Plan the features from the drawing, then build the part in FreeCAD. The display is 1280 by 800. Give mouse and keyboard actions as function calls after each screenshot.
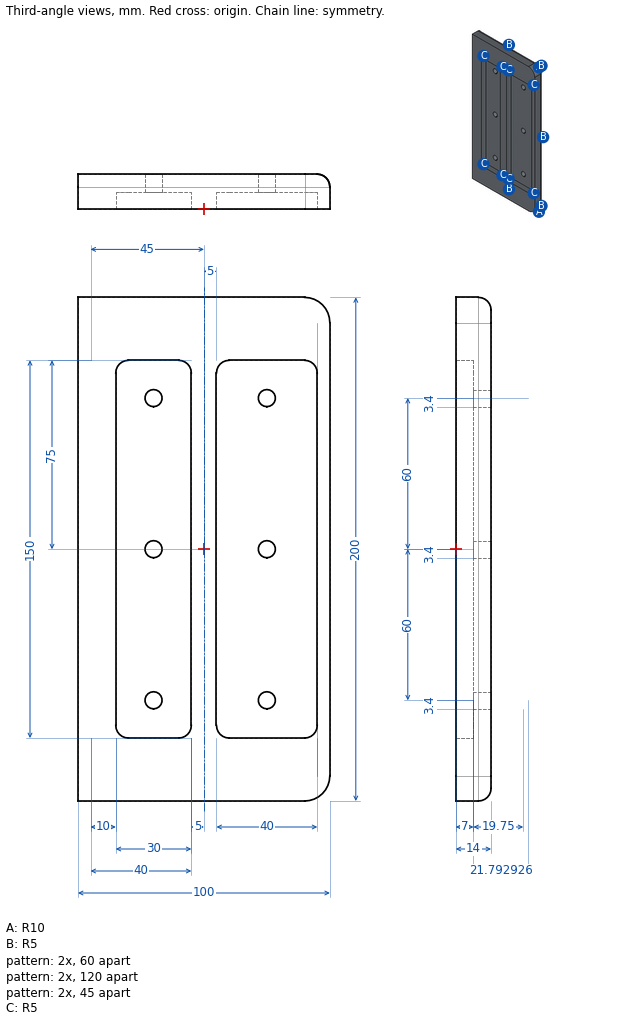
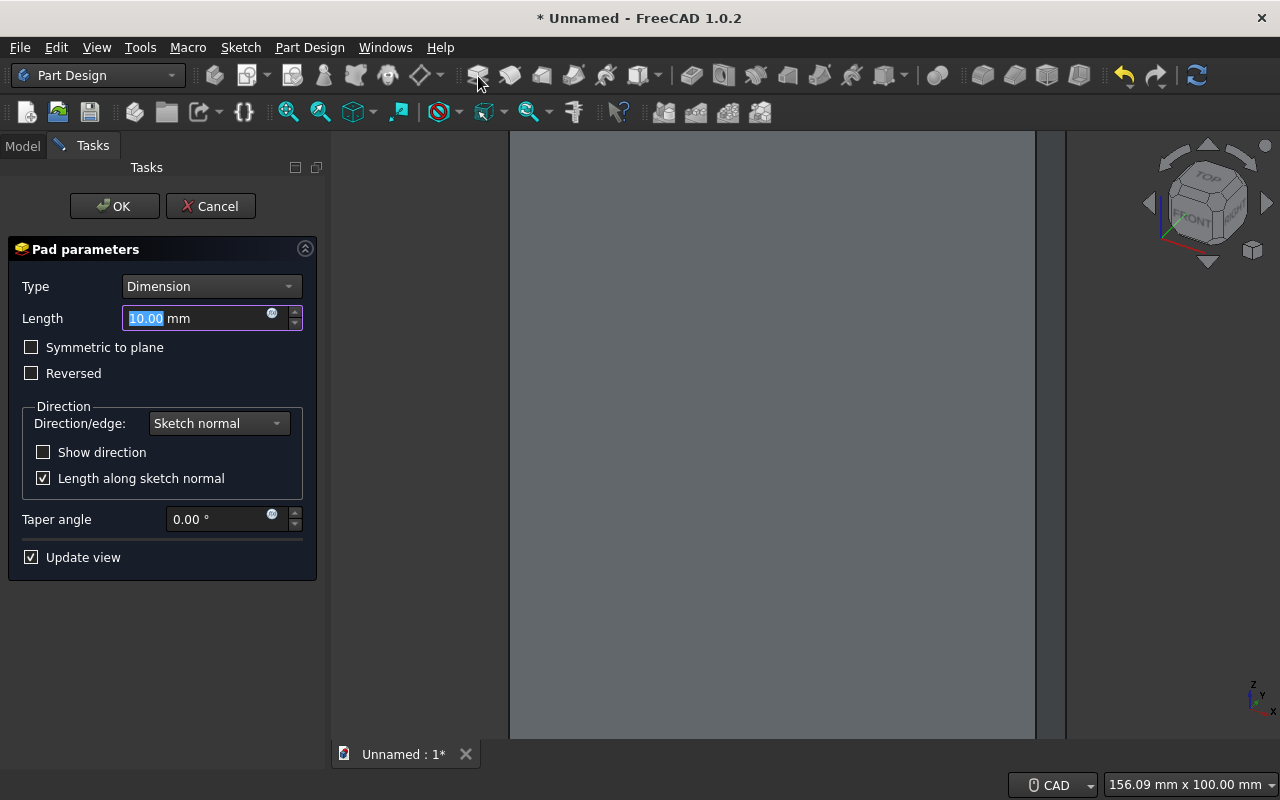
text(14)
key(Tab)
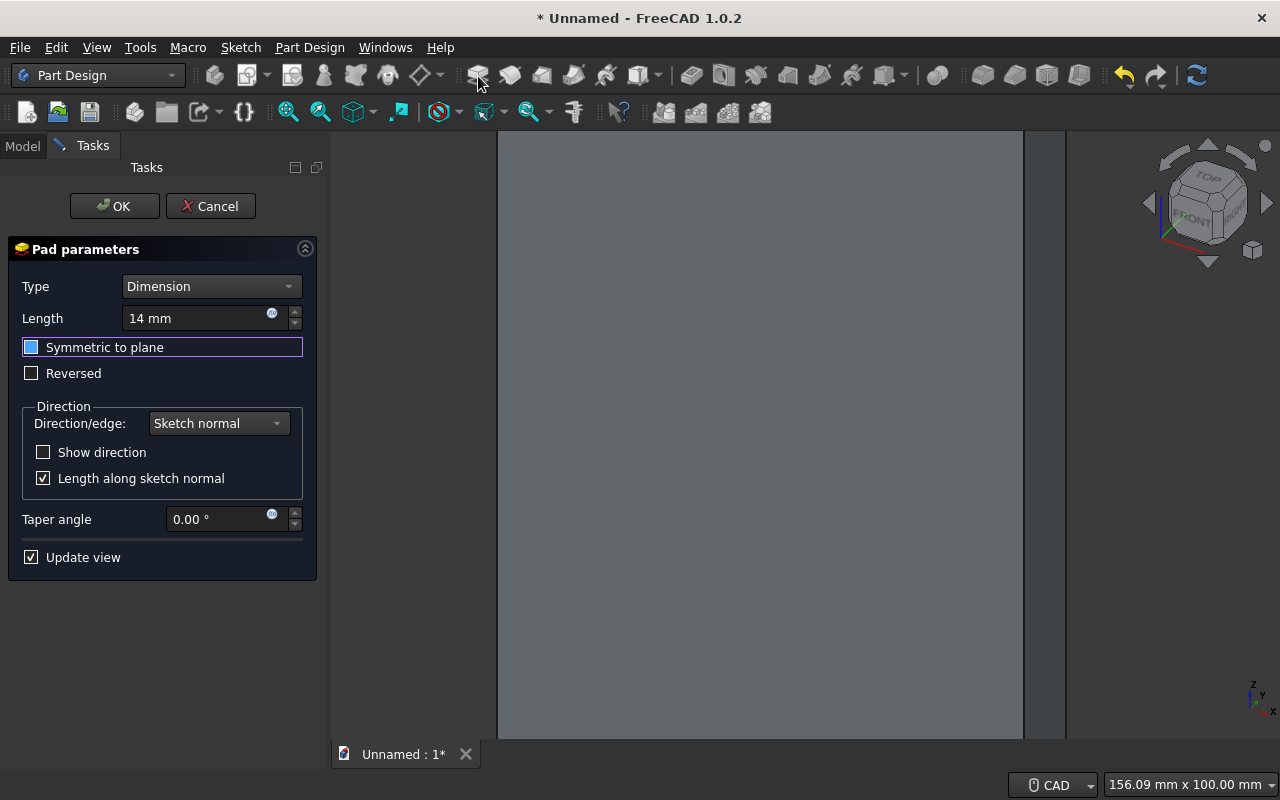
click(30, 373)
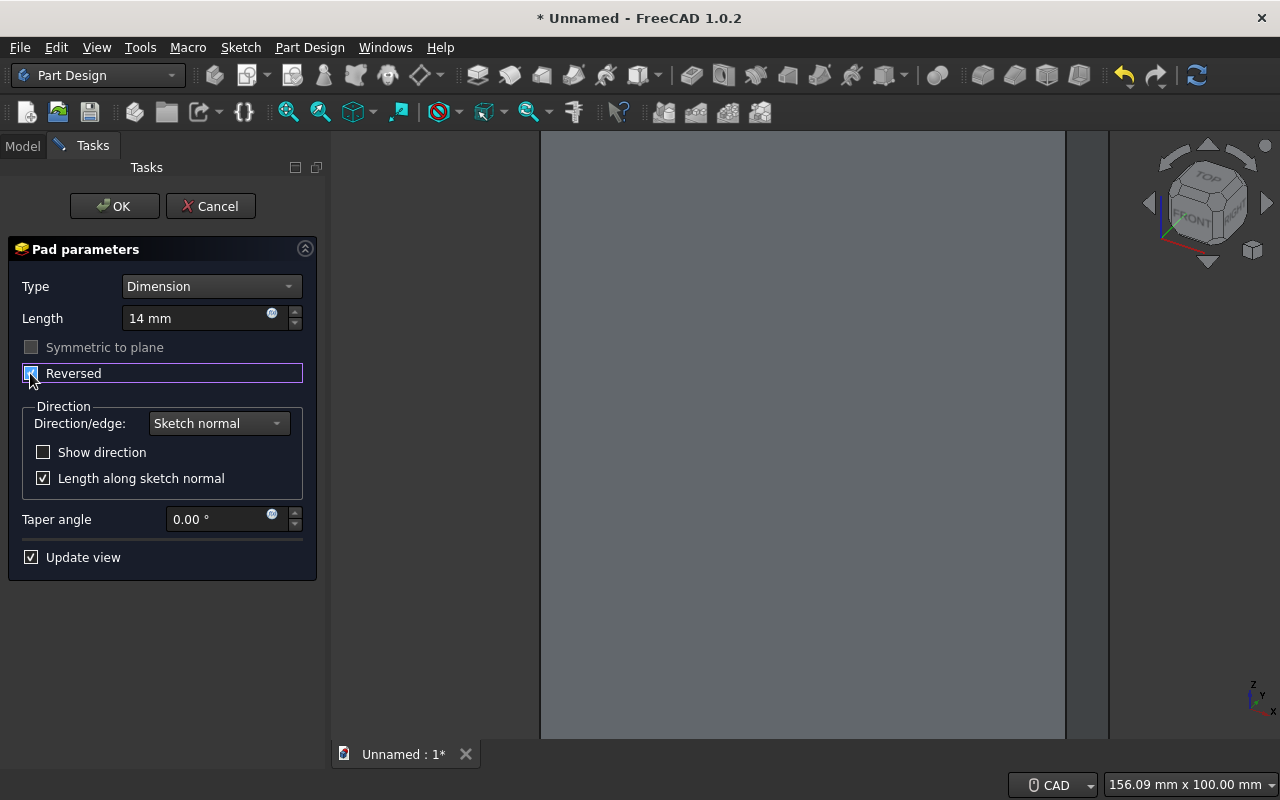
click(115, 206)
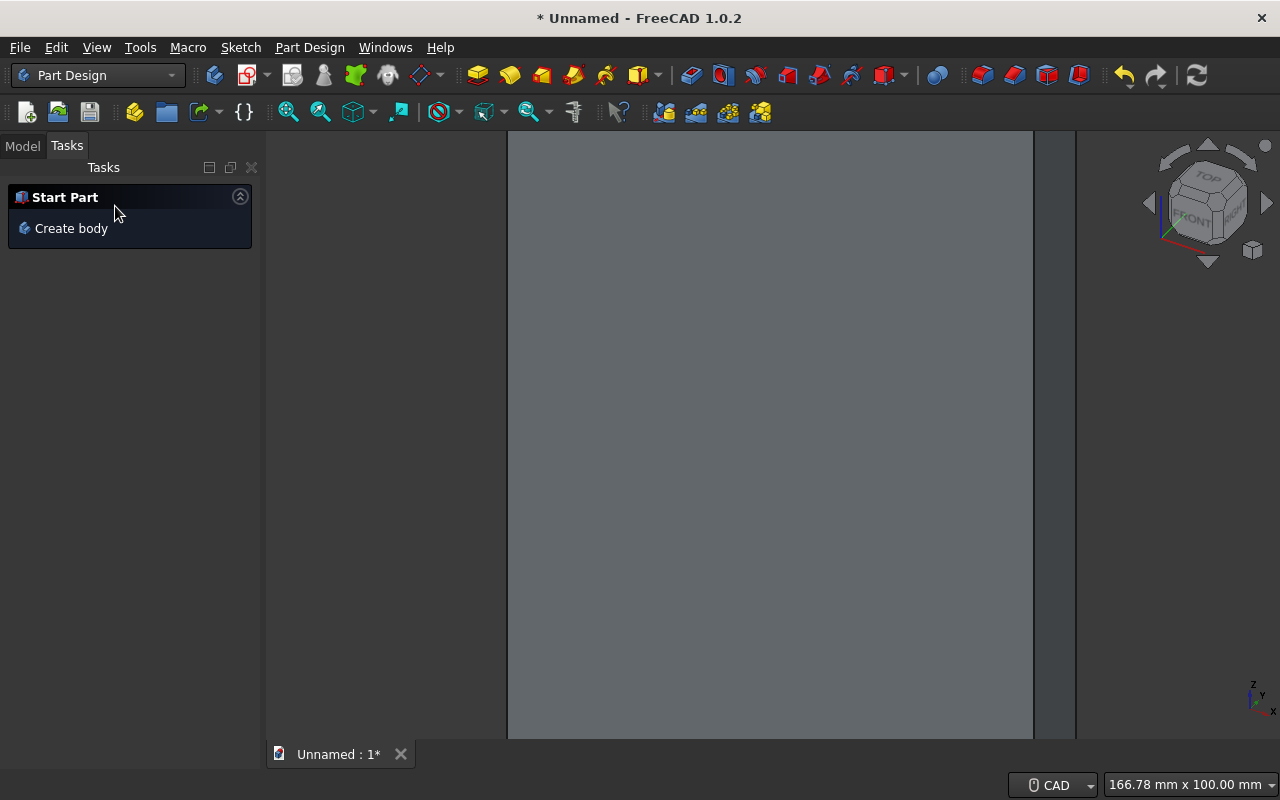
click(290, 112)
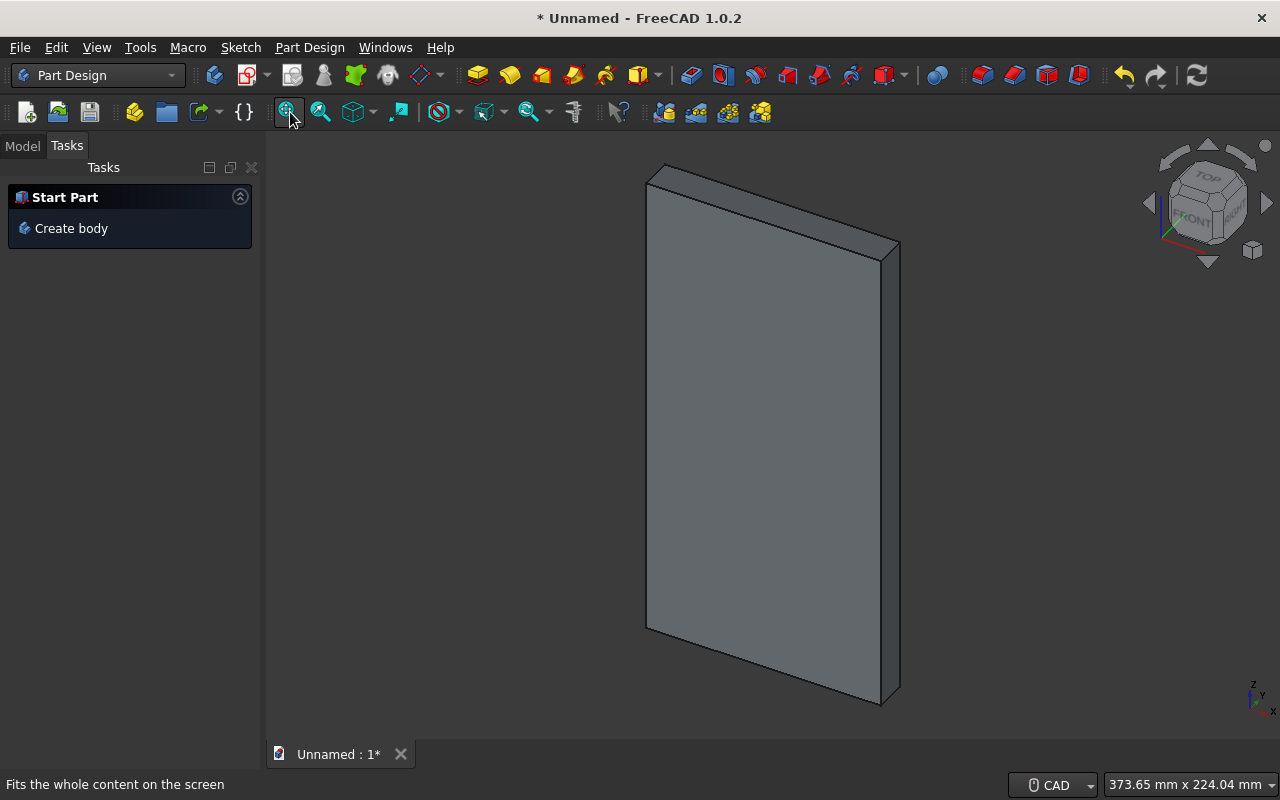
click(891, 251)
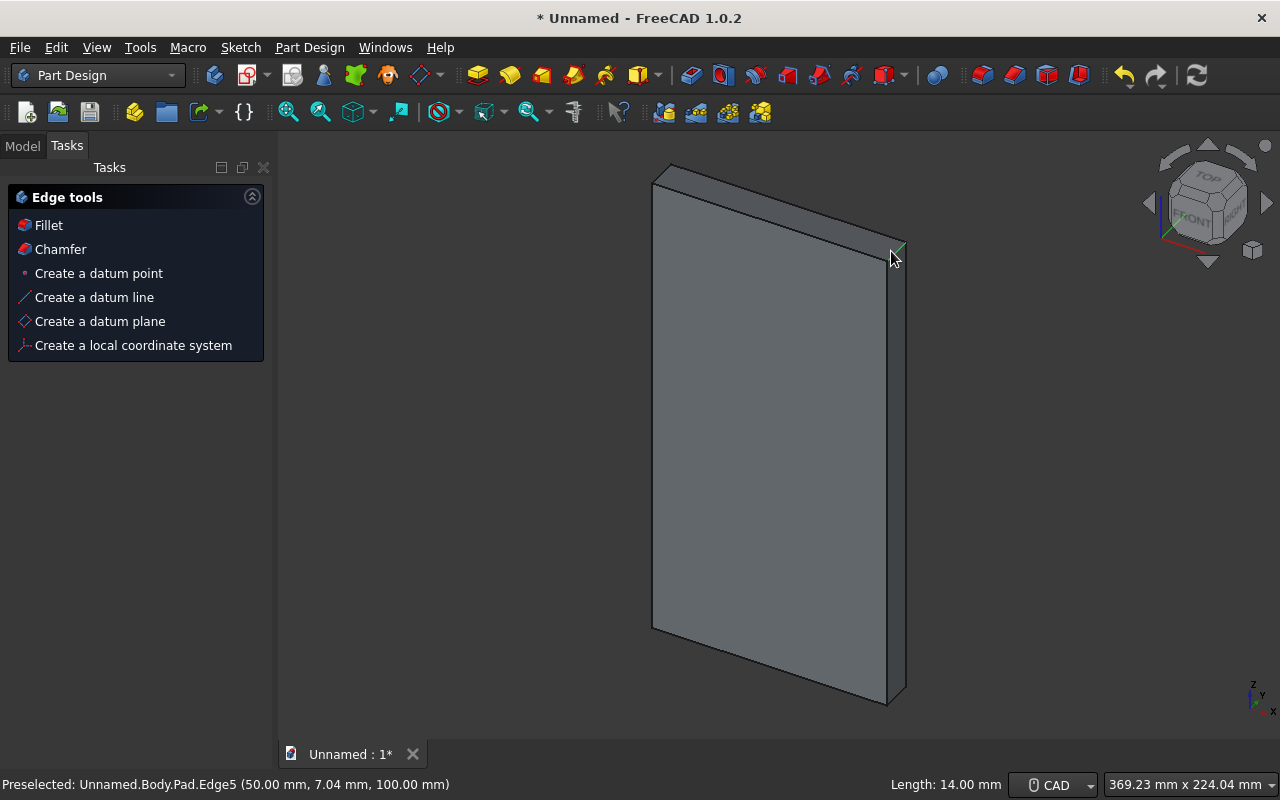
key(0)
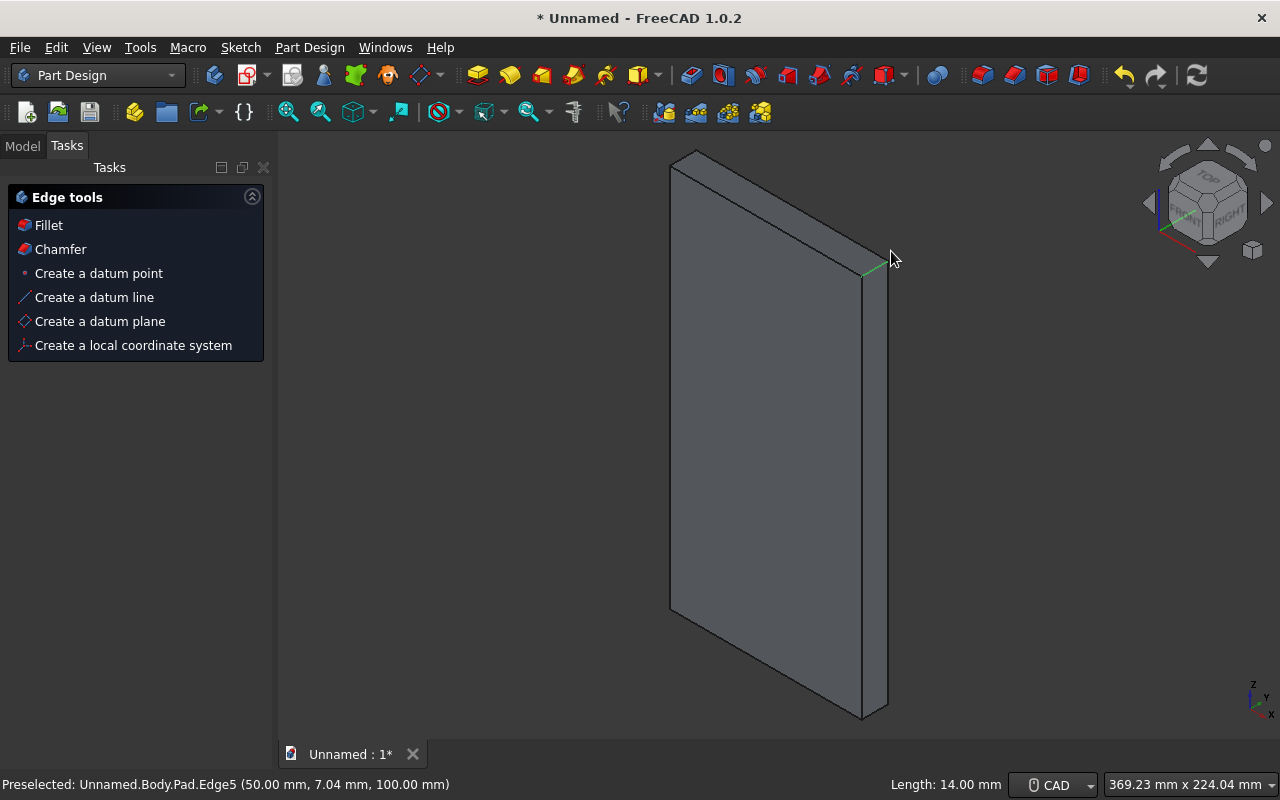
key(2)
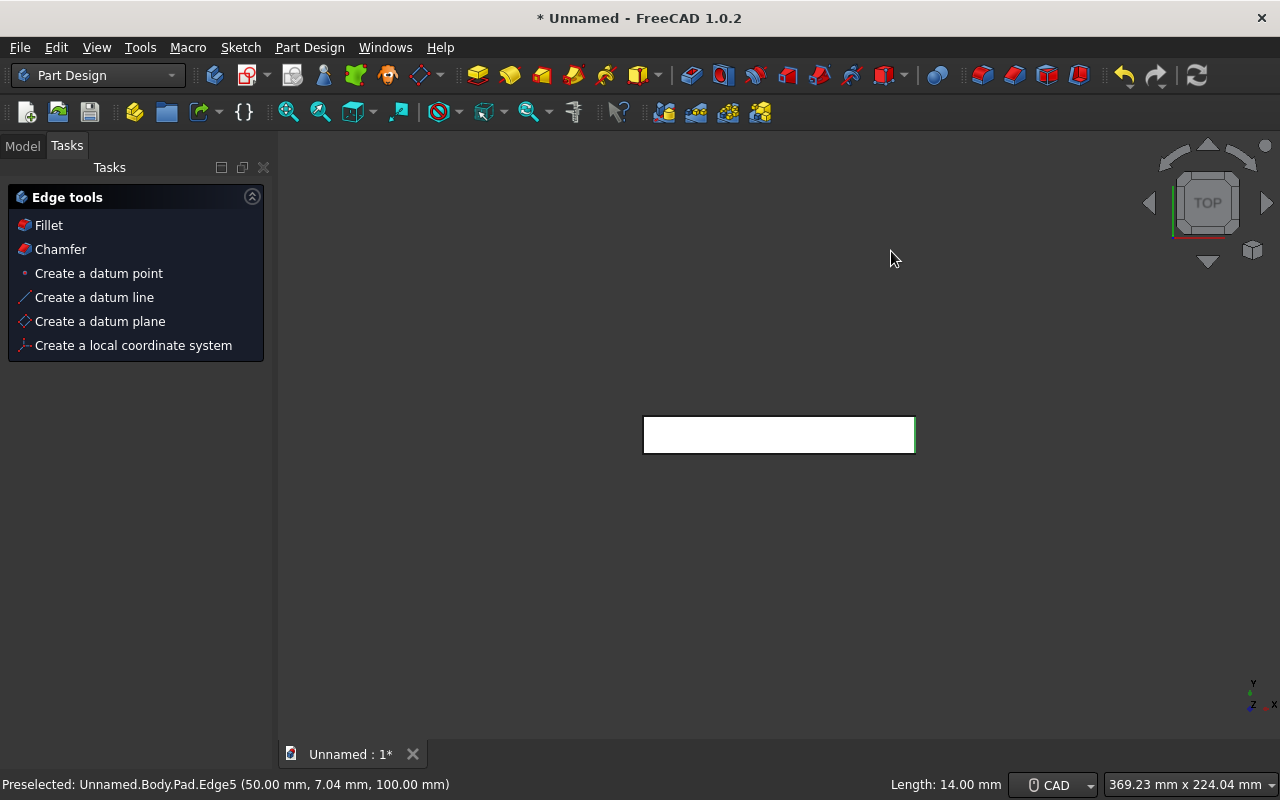
click(290, 112)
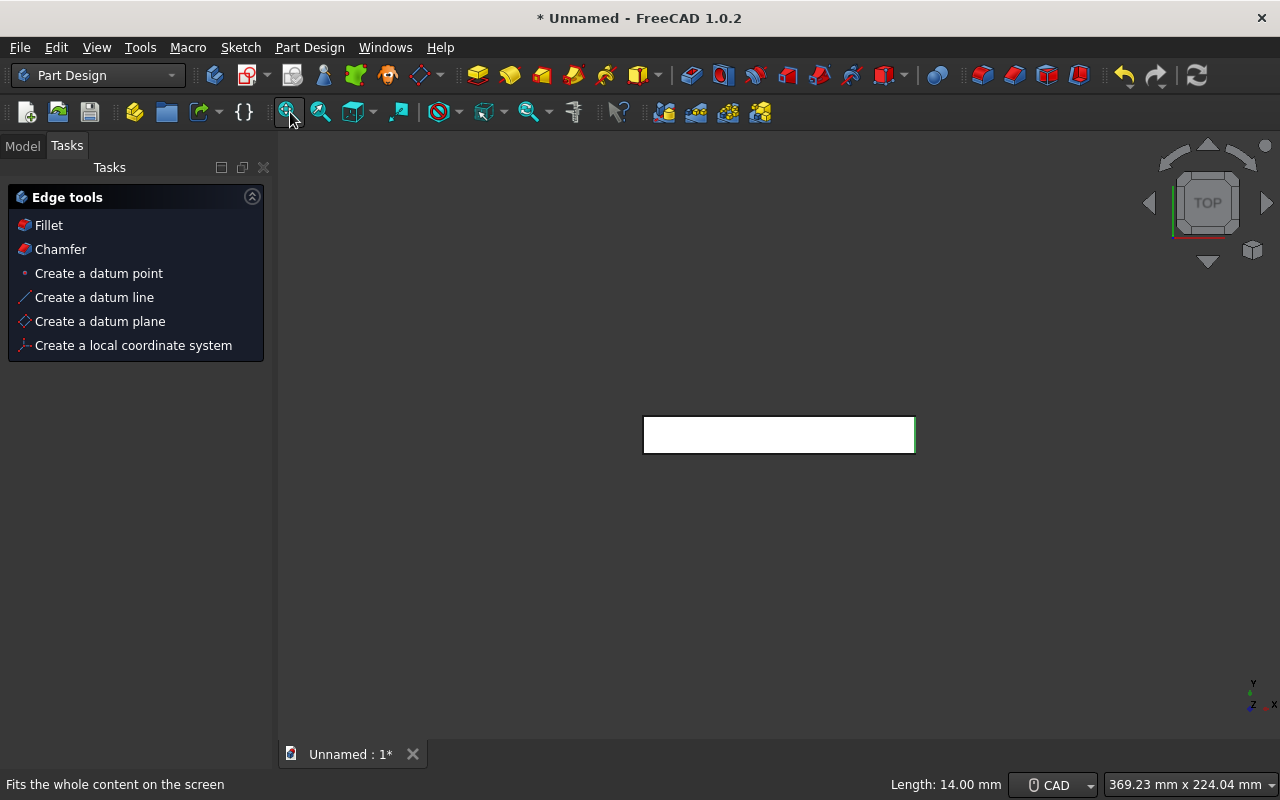
key(1)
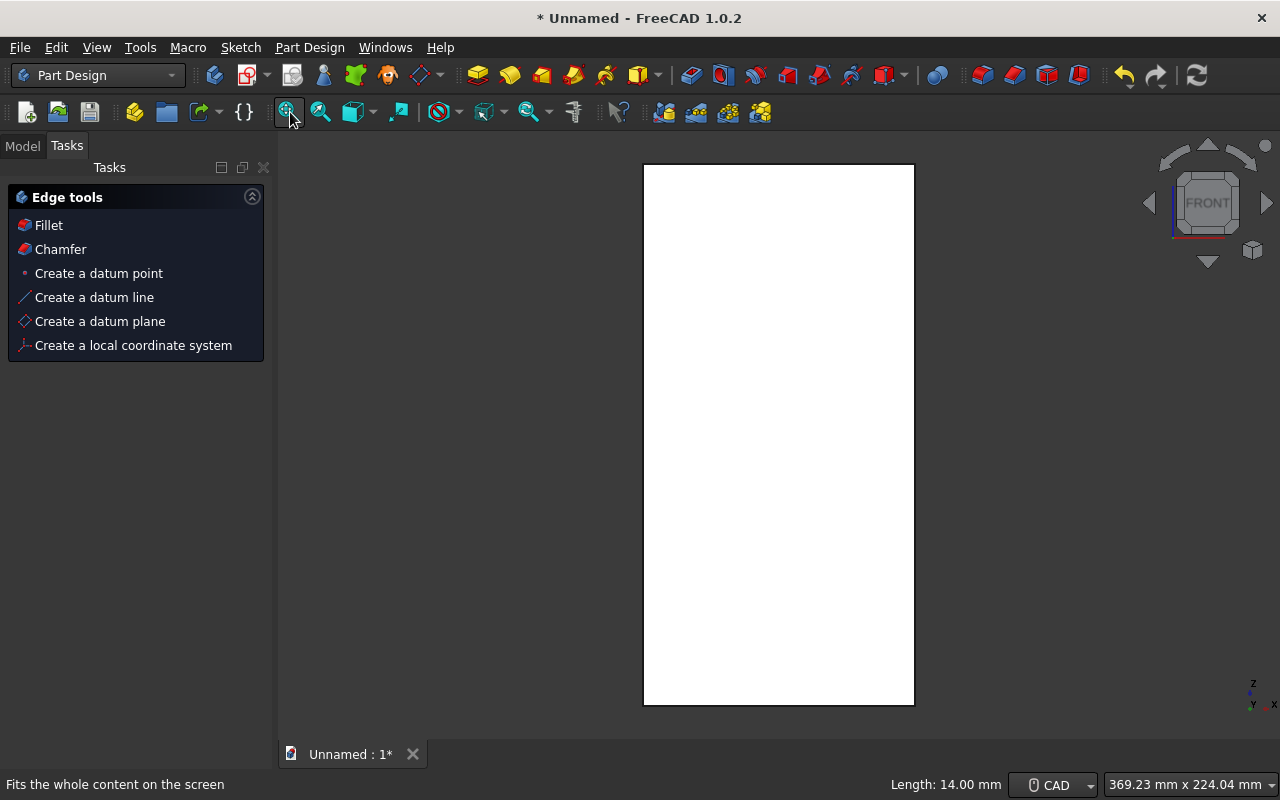
key(3)